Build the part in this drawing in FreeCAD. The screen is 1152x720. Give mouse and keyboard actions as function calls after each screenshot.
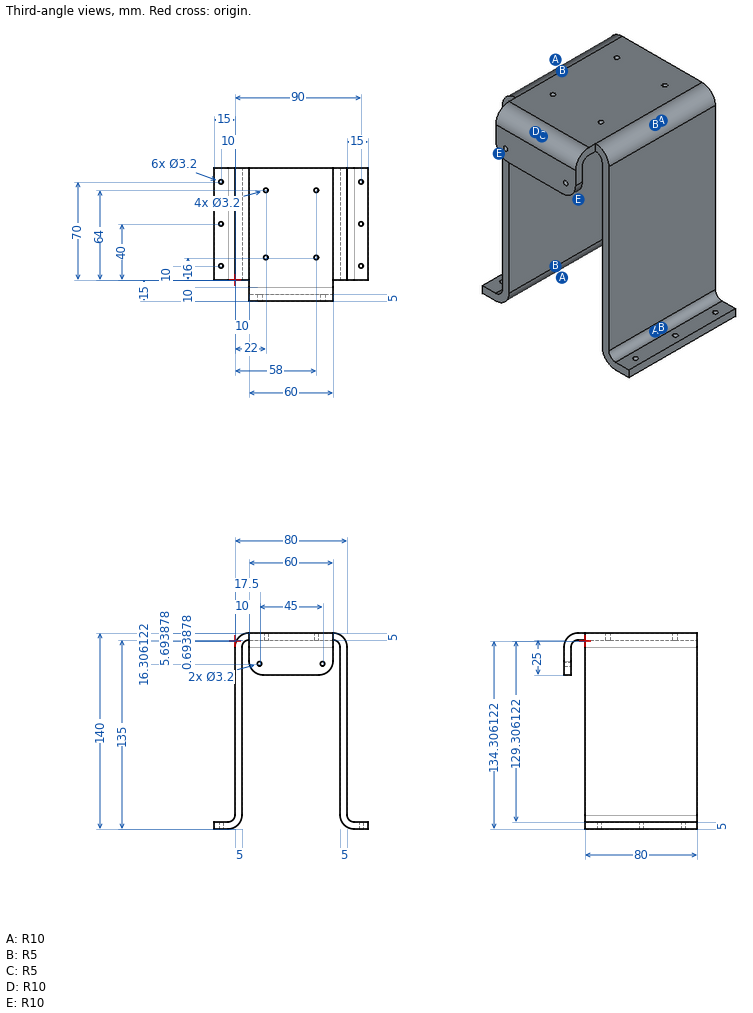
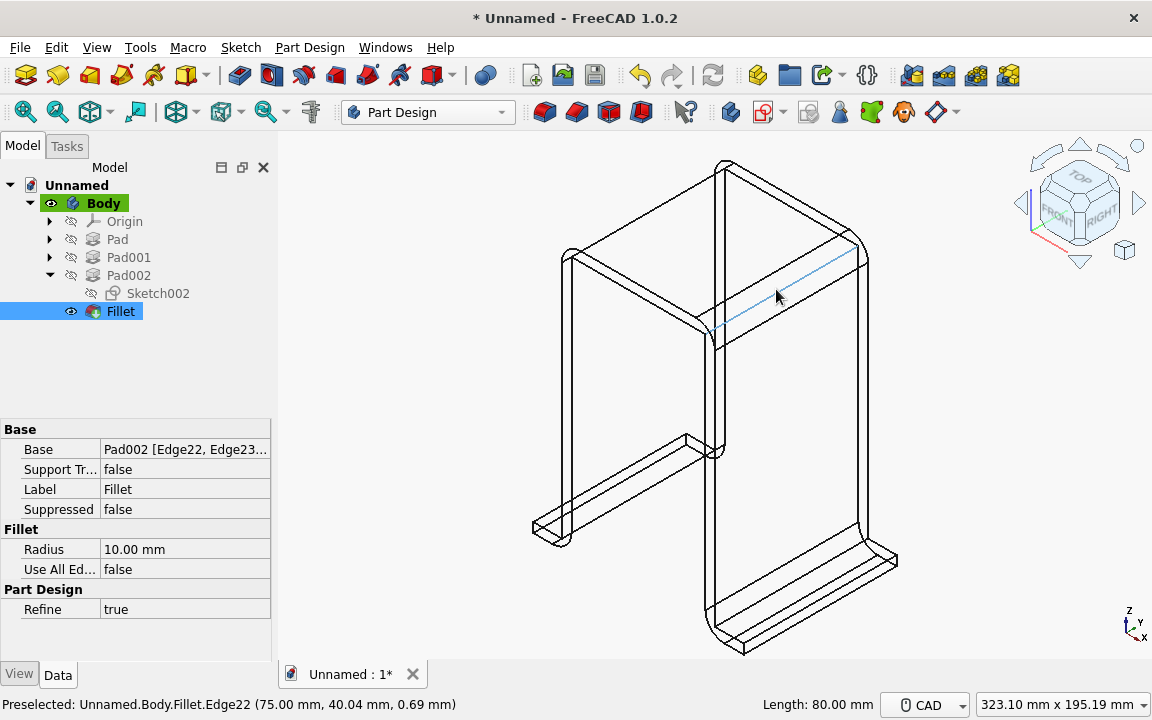
click(792, 582, ctrl)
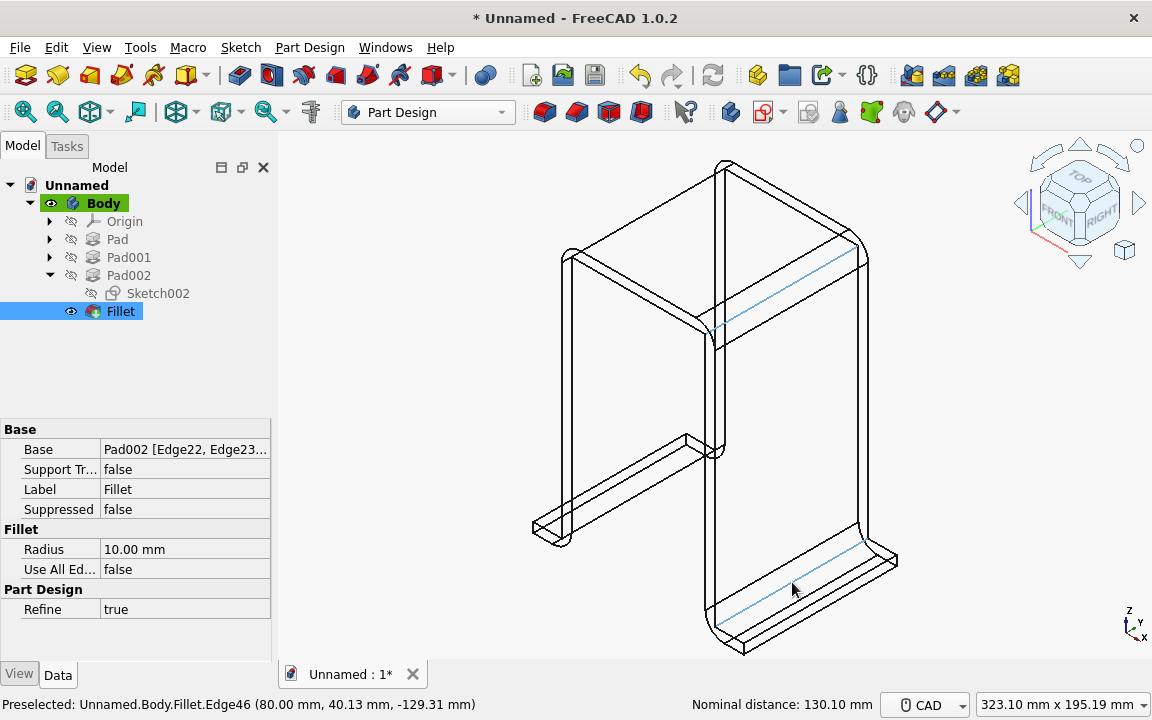
key(2)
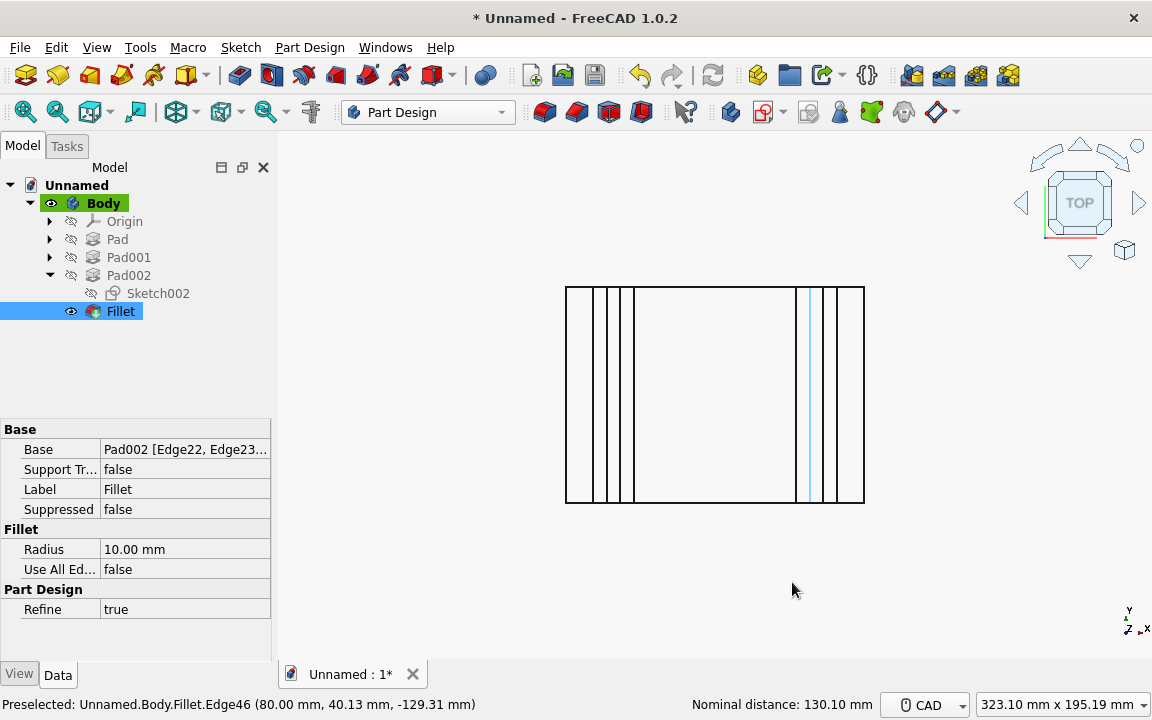
click(26, 112)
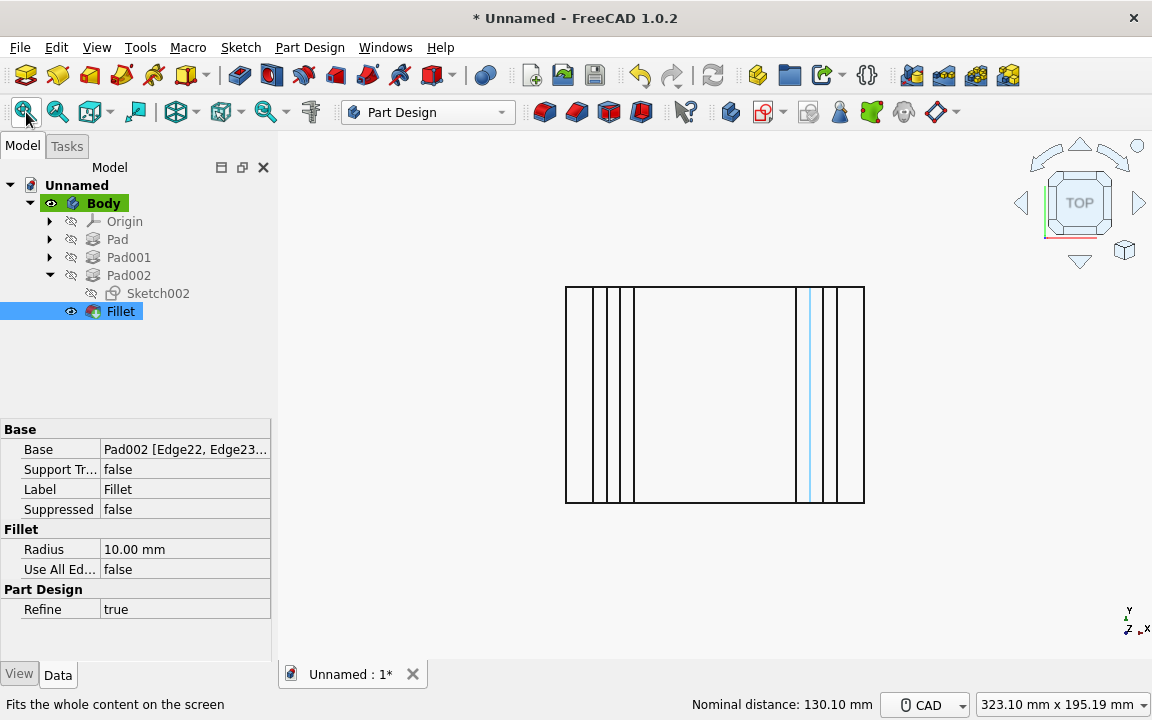
click(620, 394, ctrl)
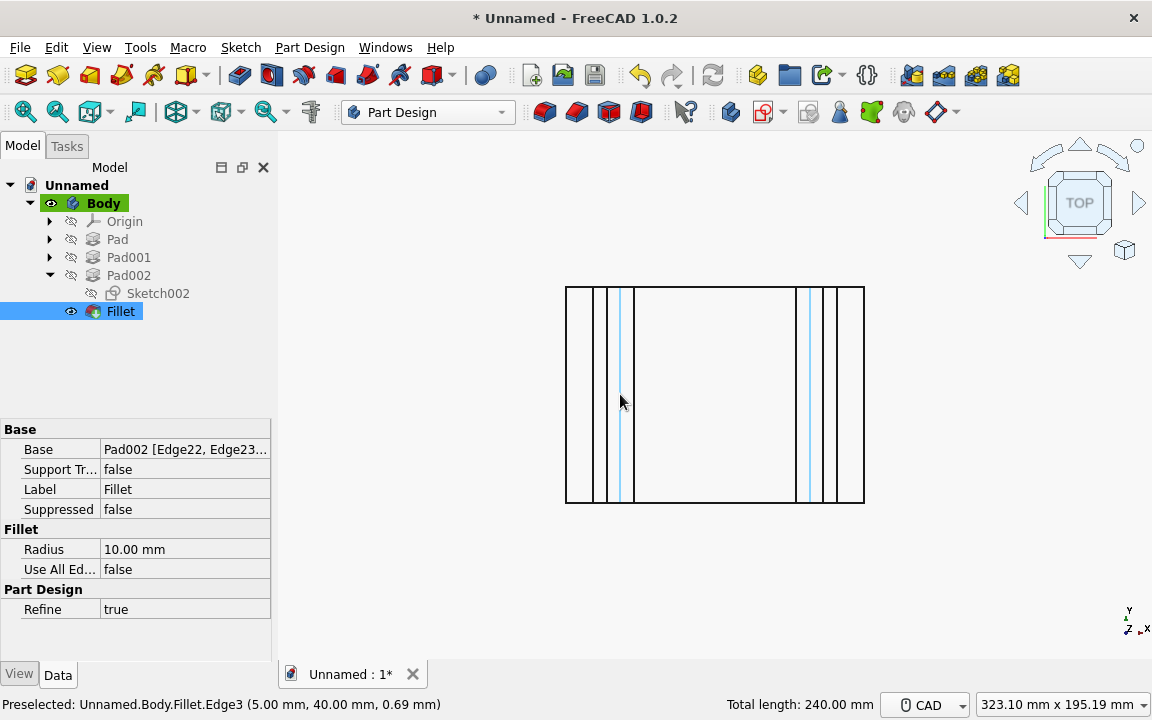
key(1)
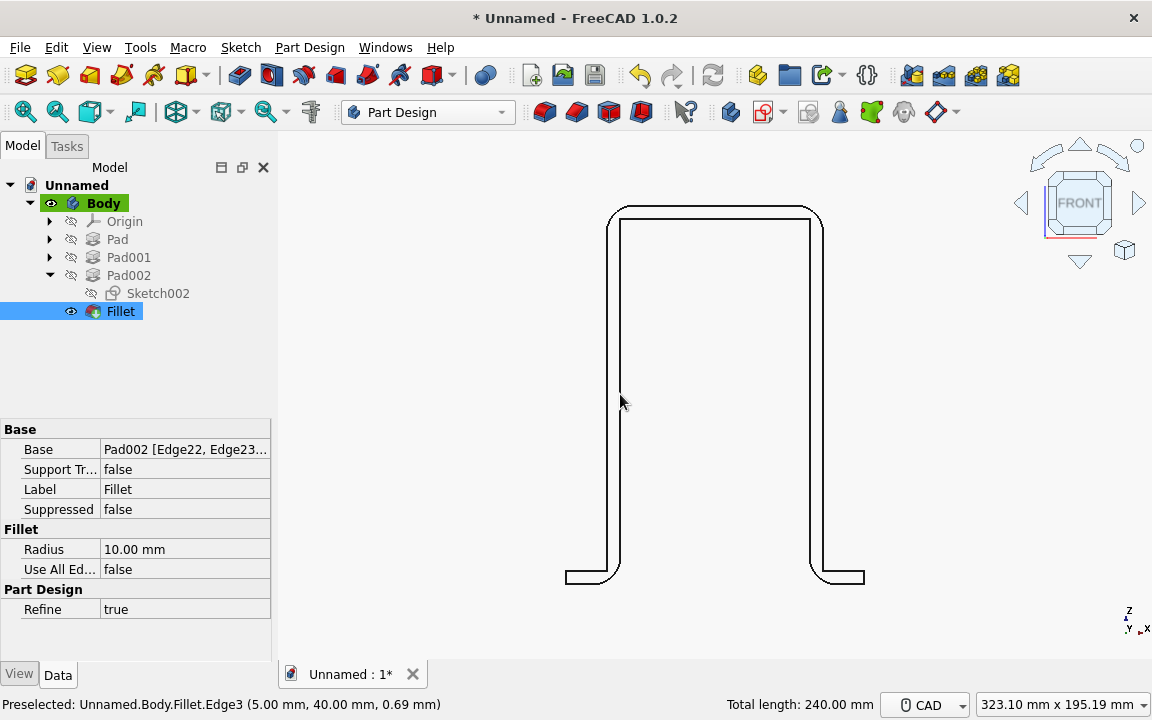
key(3)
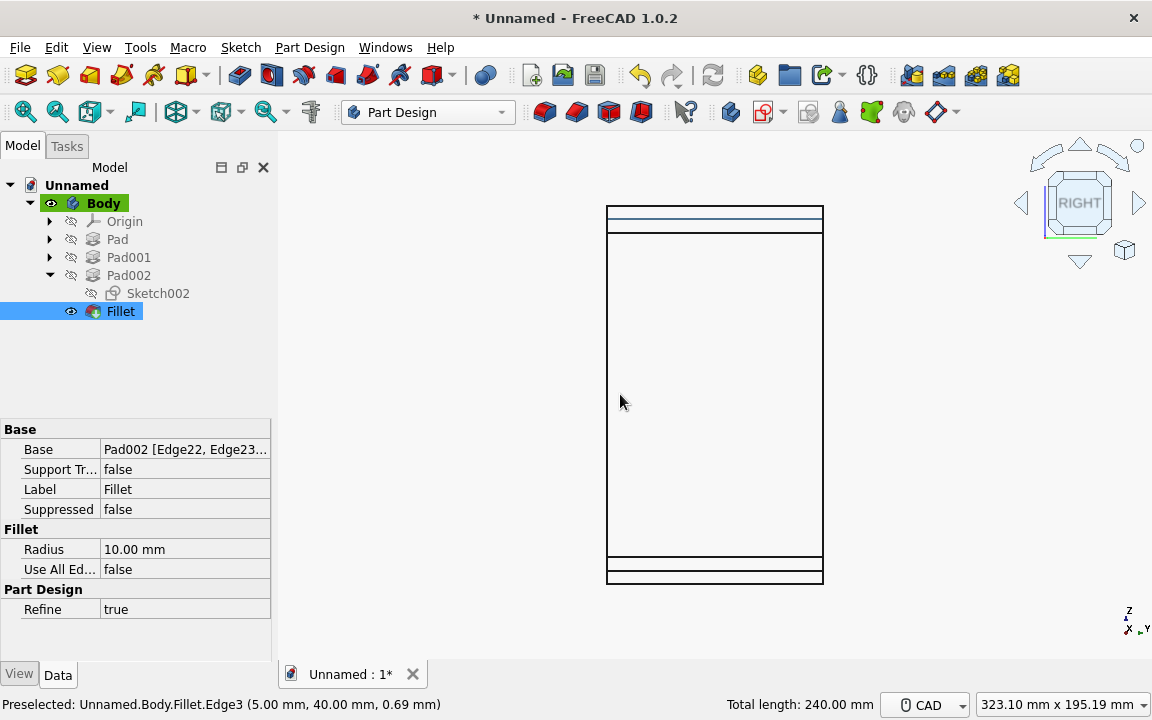
key(5)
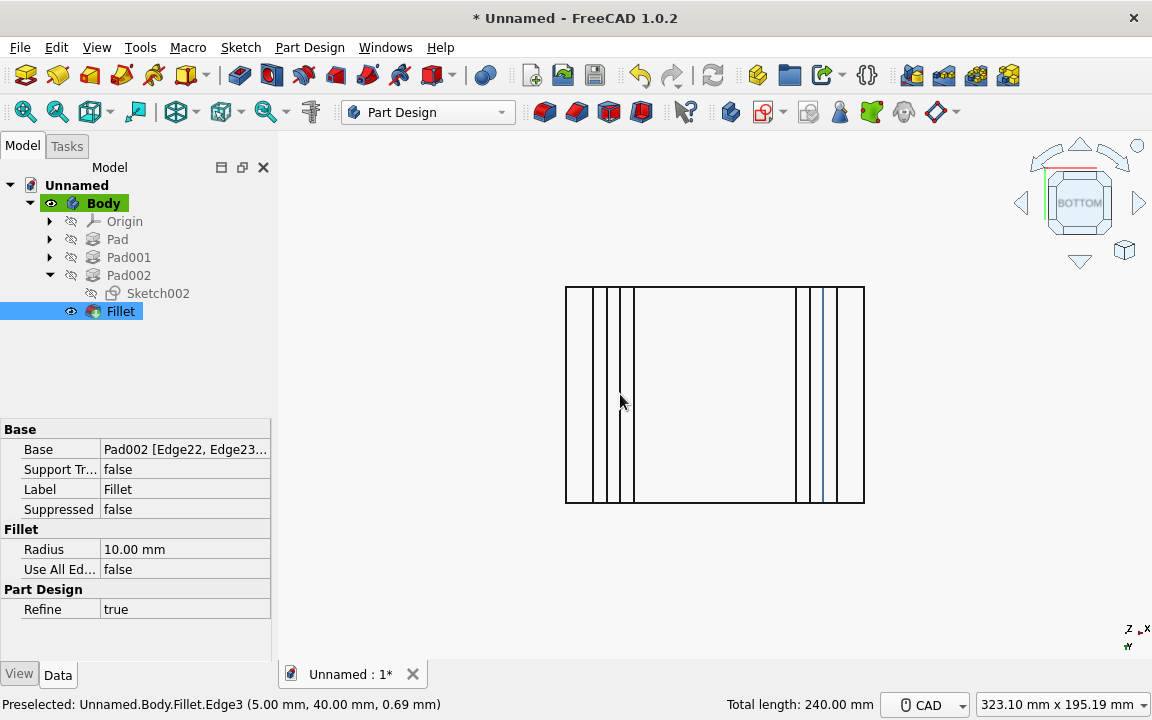
click(26, 112)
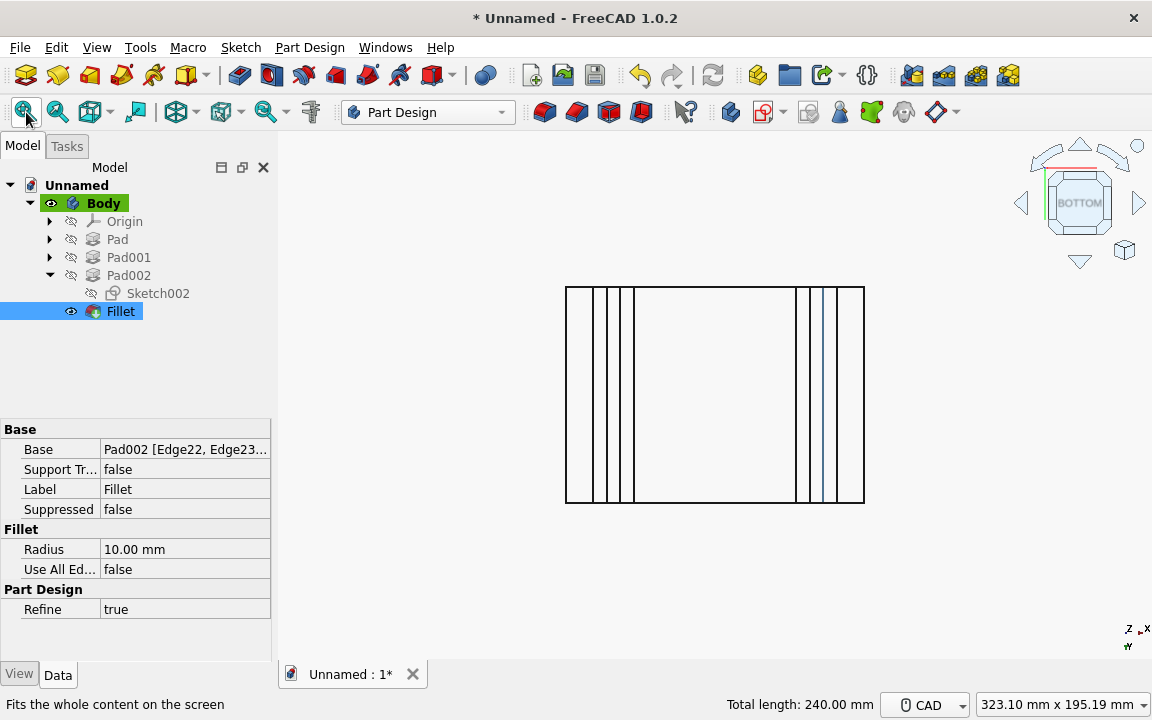
click(607, 394, ctrl)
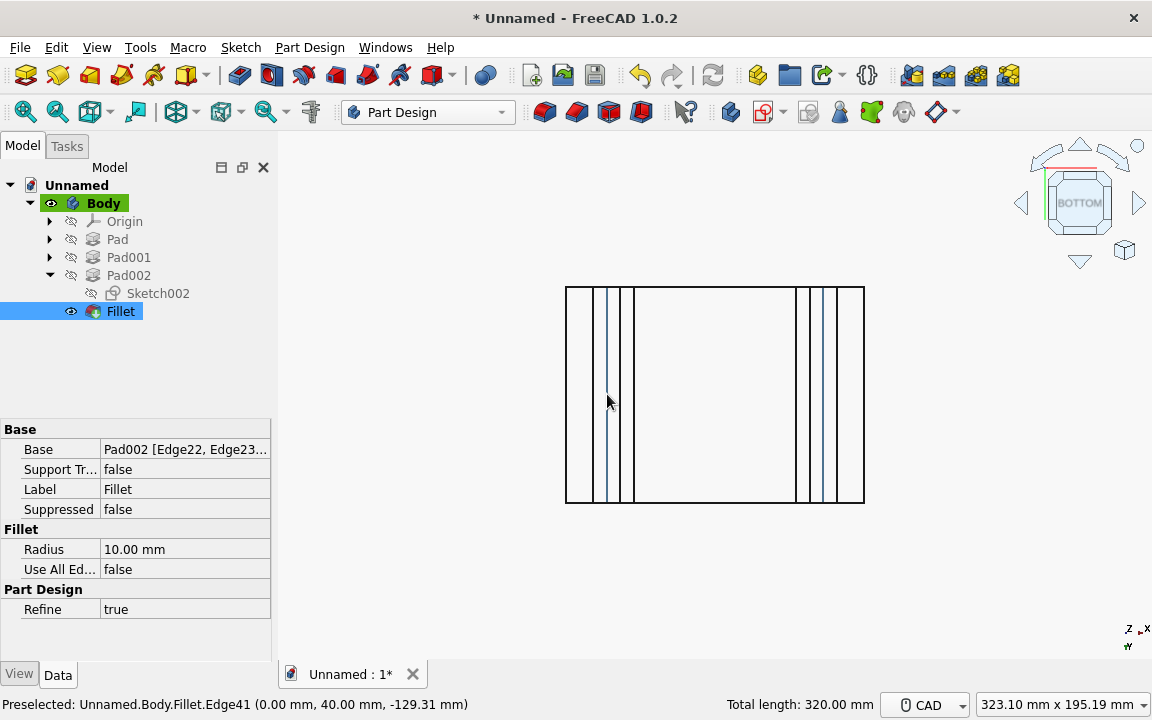
key(v)
key(1)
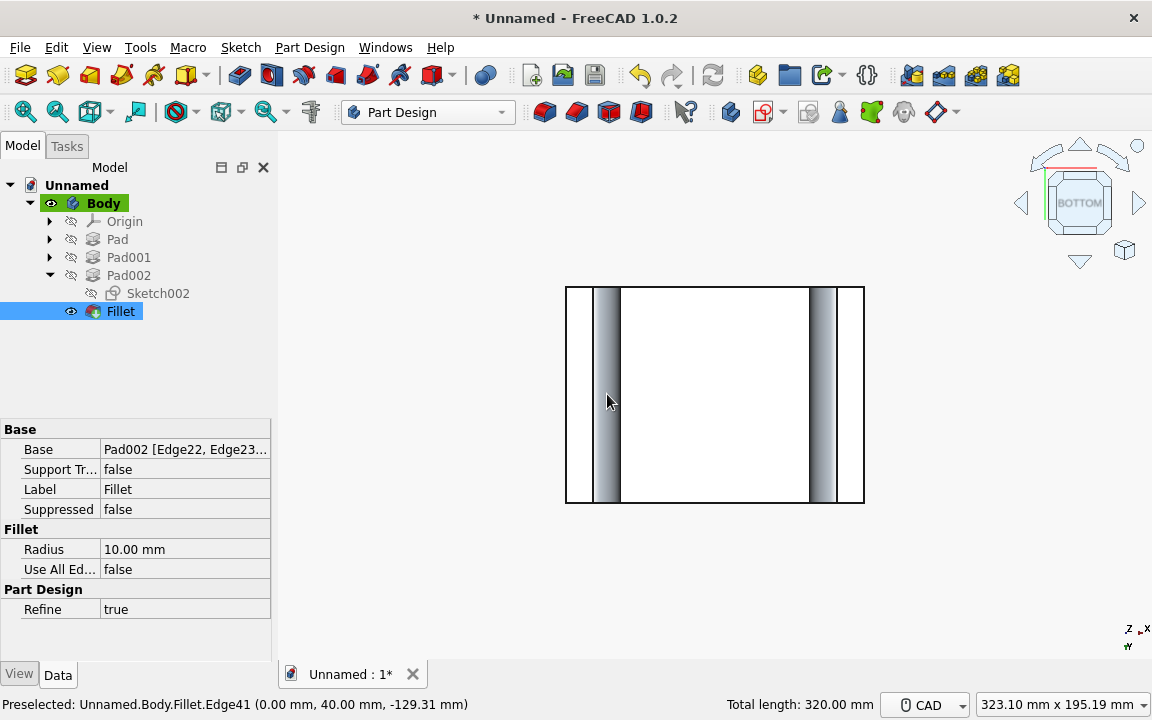
click(546, 112)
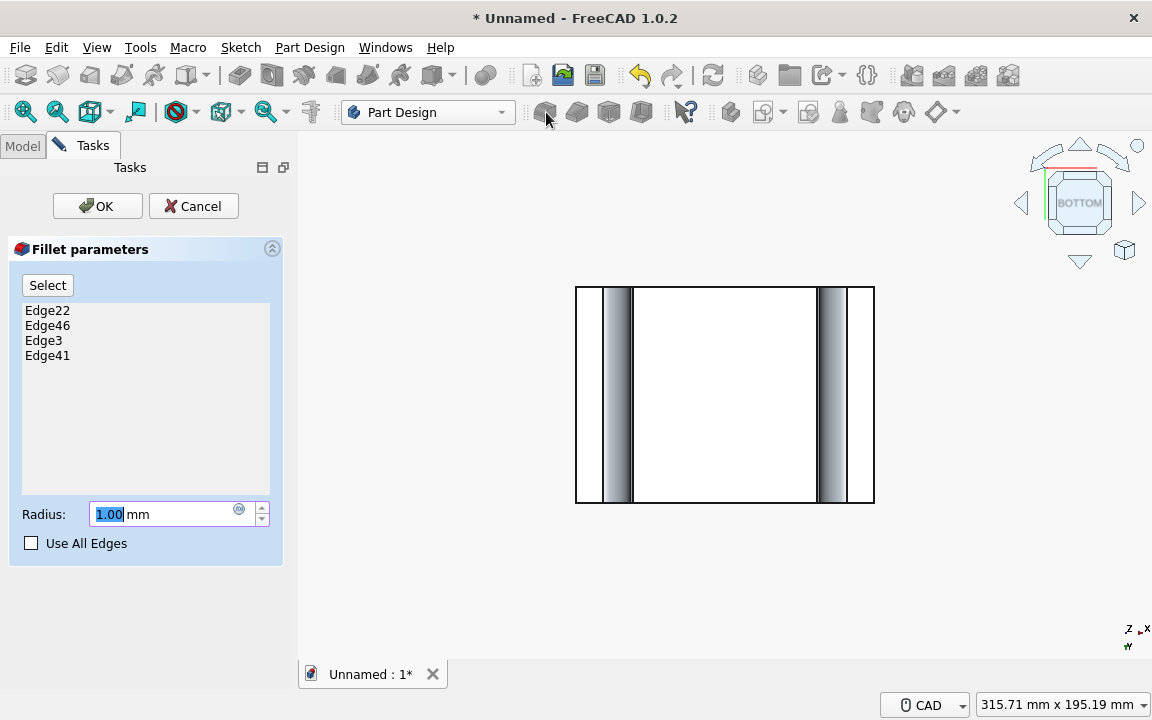
text(5)
key(Tab)